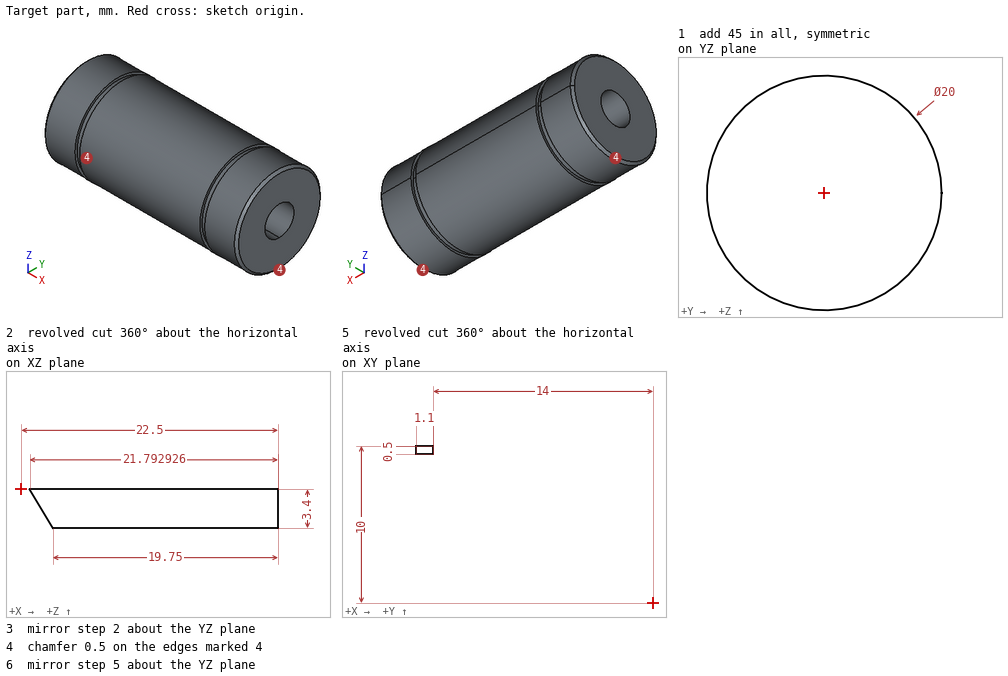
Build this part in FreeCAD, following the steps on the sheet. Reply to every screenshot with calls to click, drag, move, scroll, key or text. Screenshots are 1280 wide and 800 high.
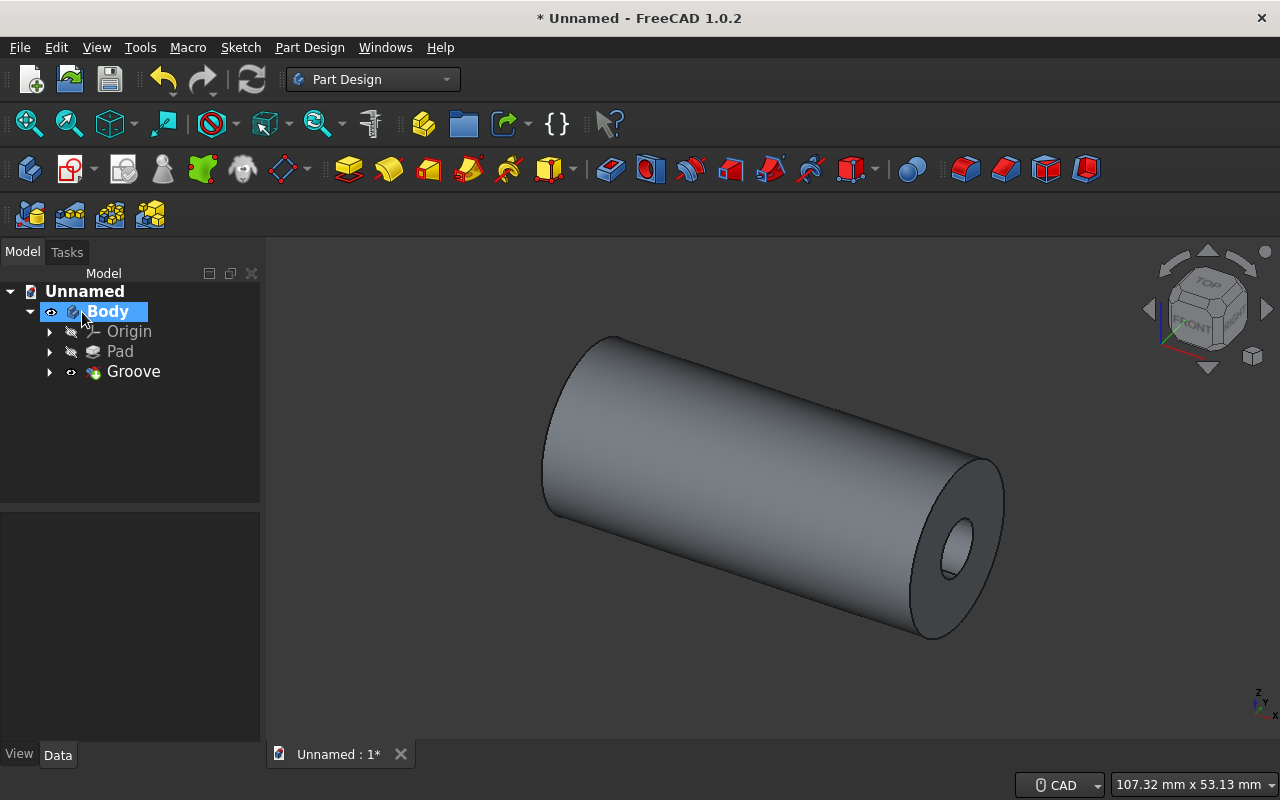
click(116, 372)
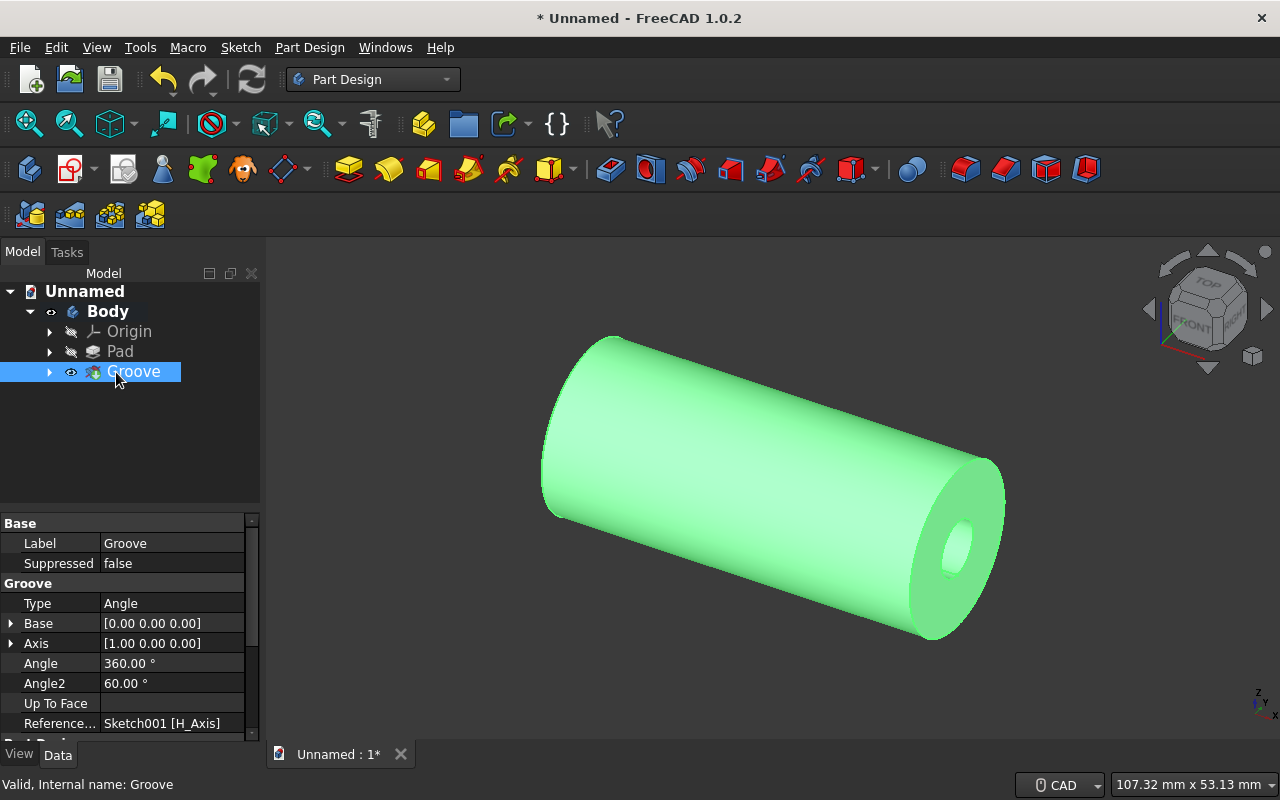
click(30, 214)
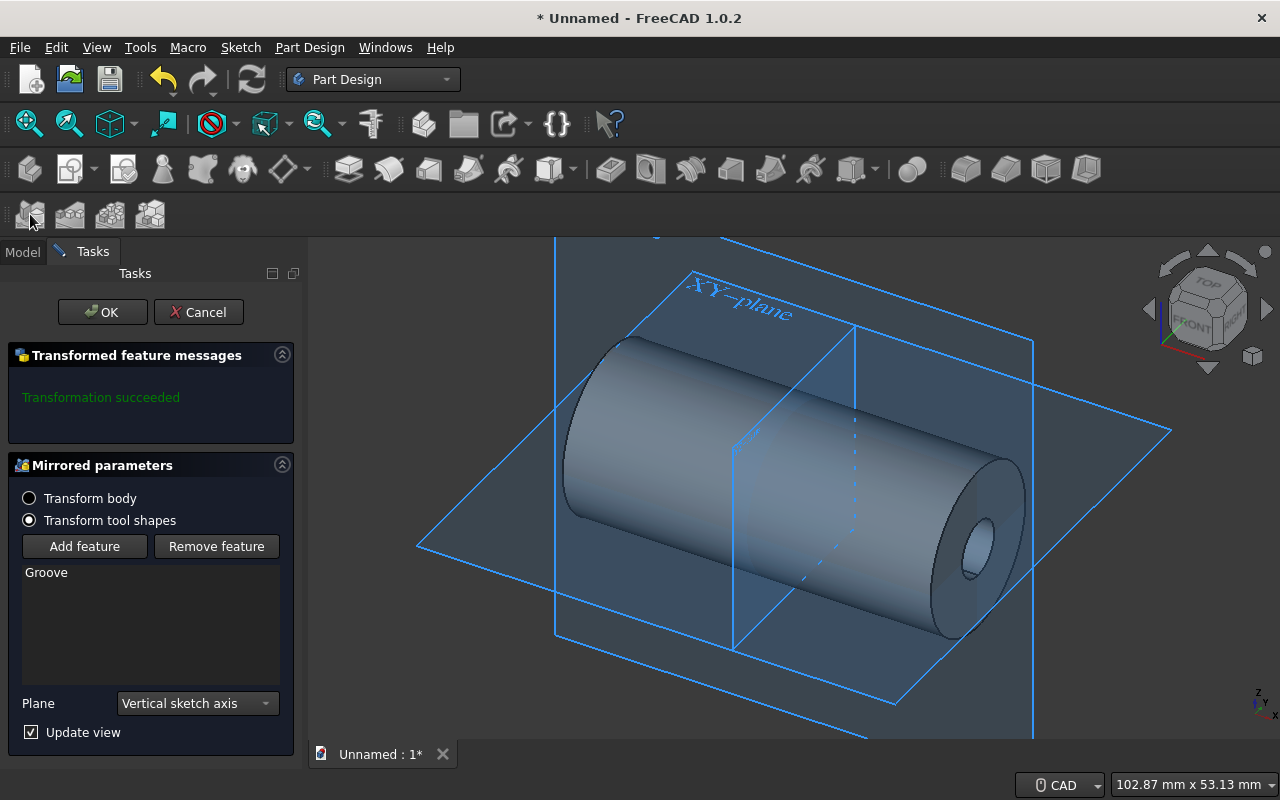
click(198, 704)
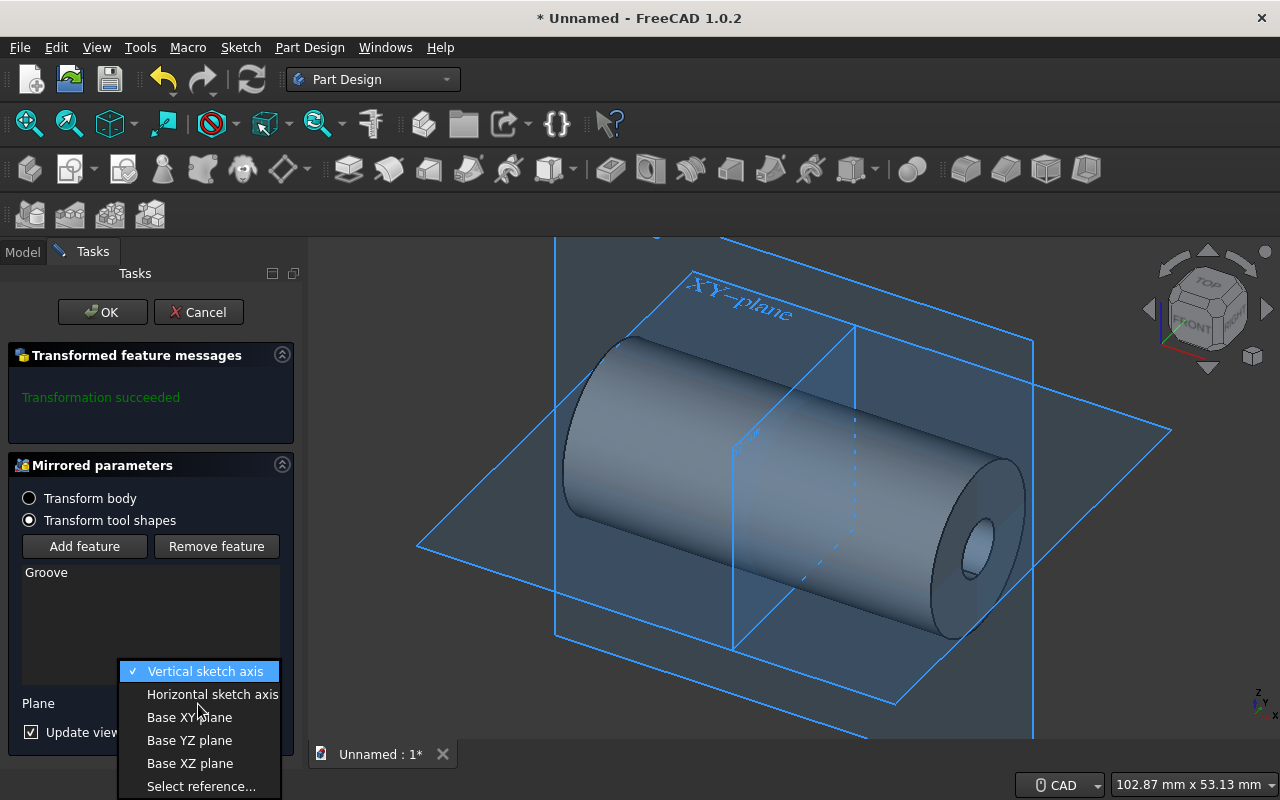
click(198, 740)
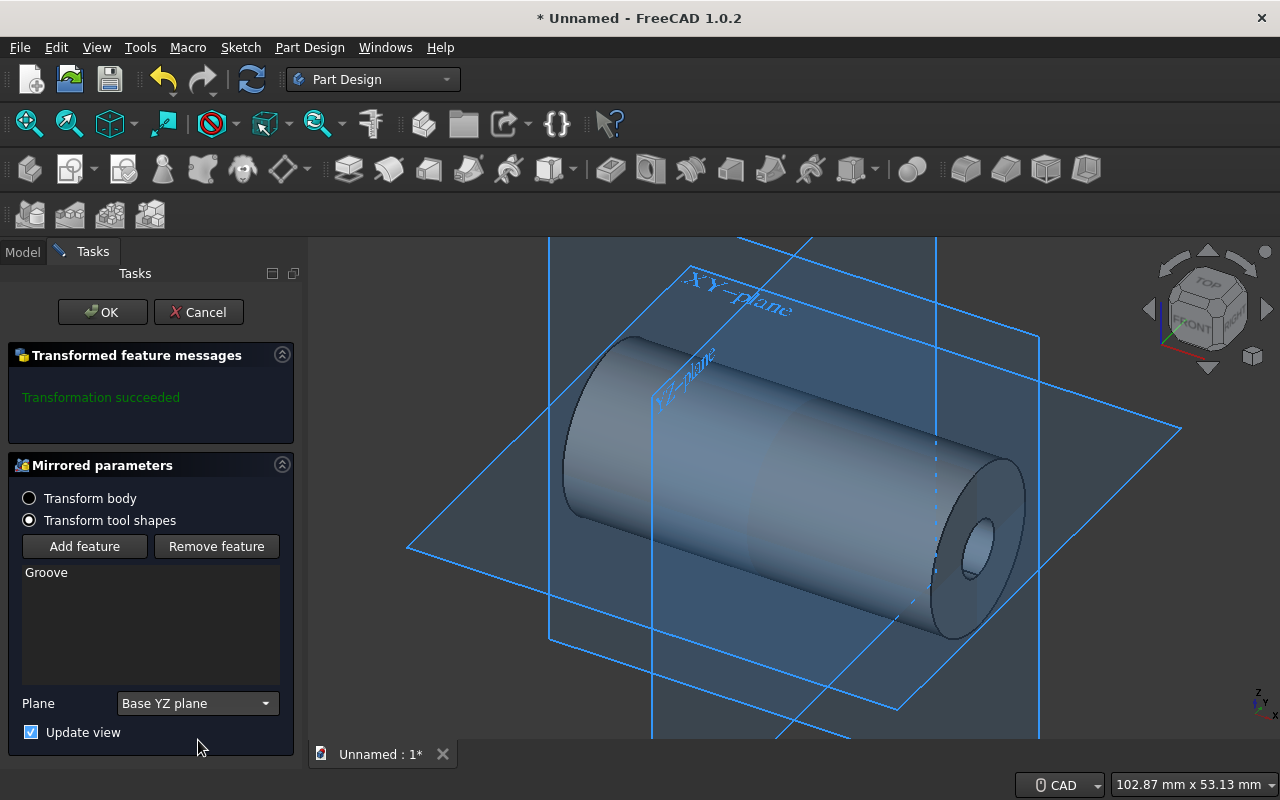
click(103, 312)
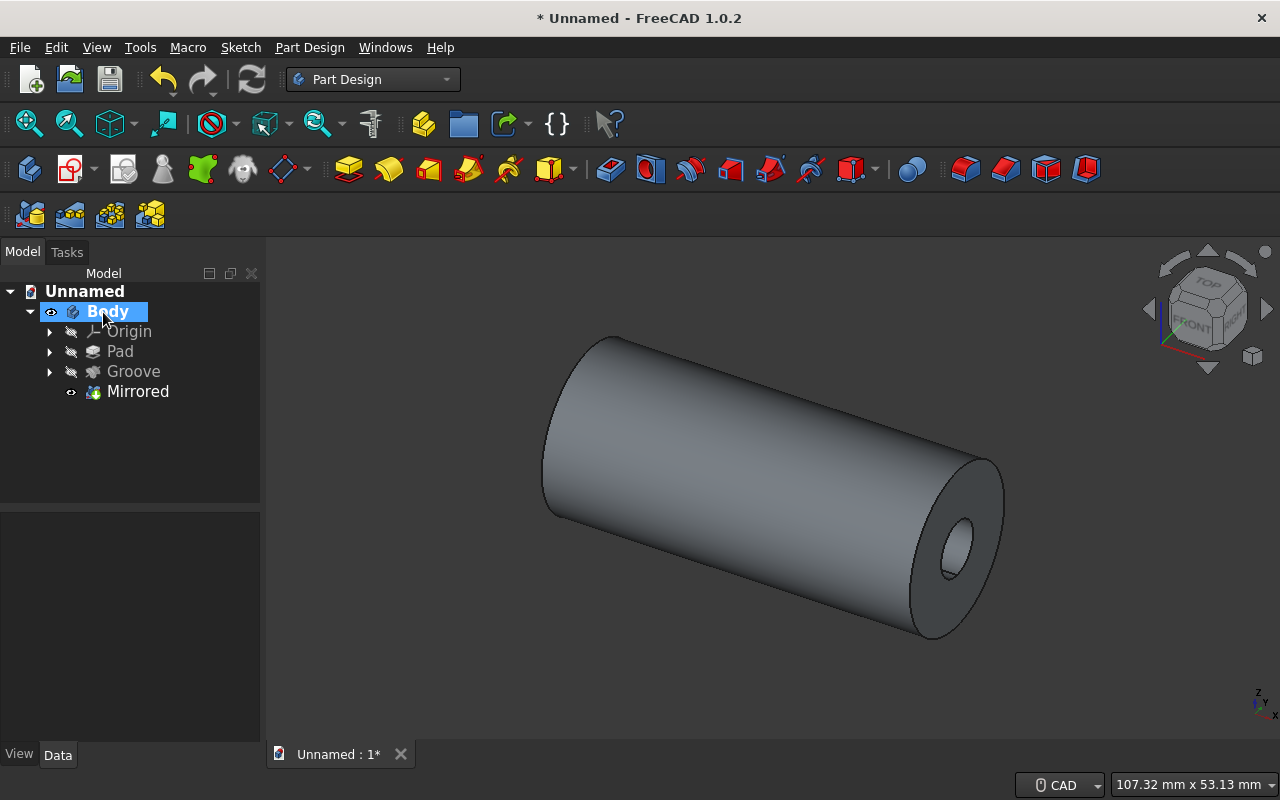
click(574, 367)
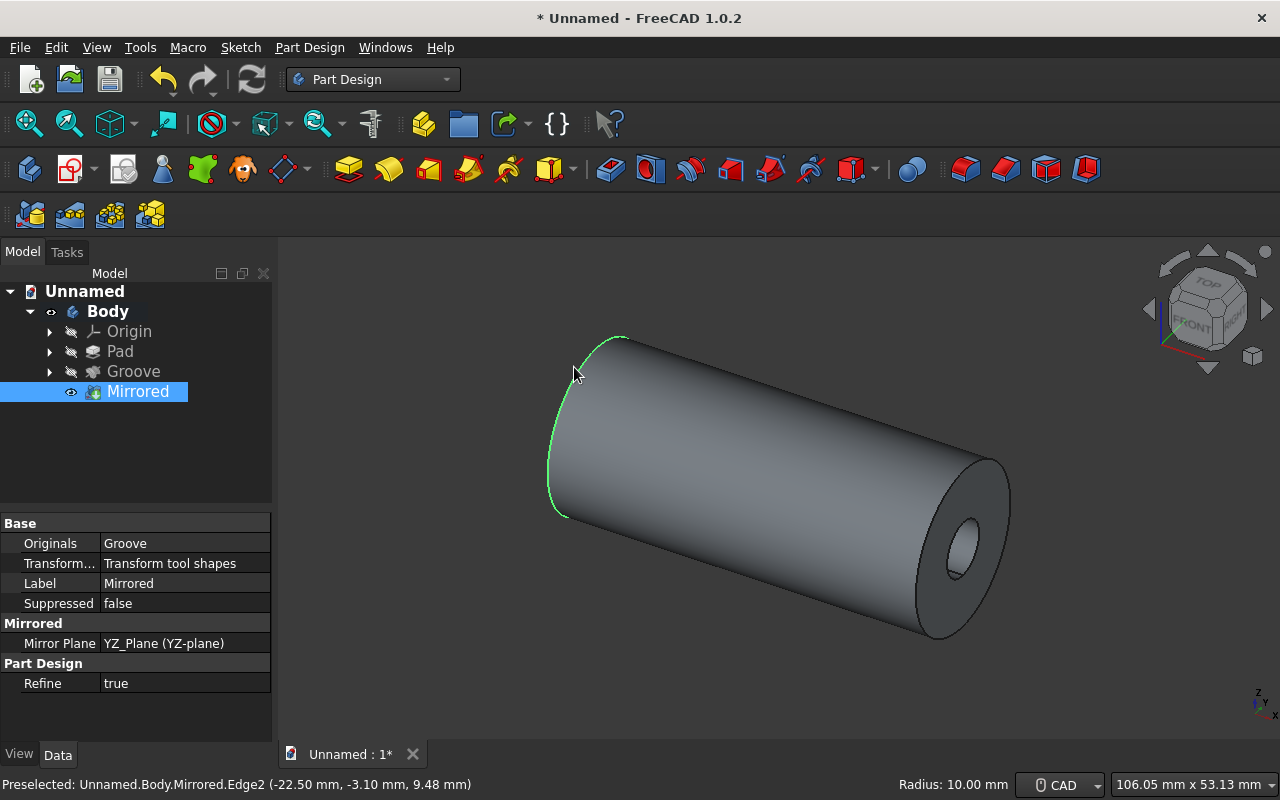
click(916, 595, ctrl)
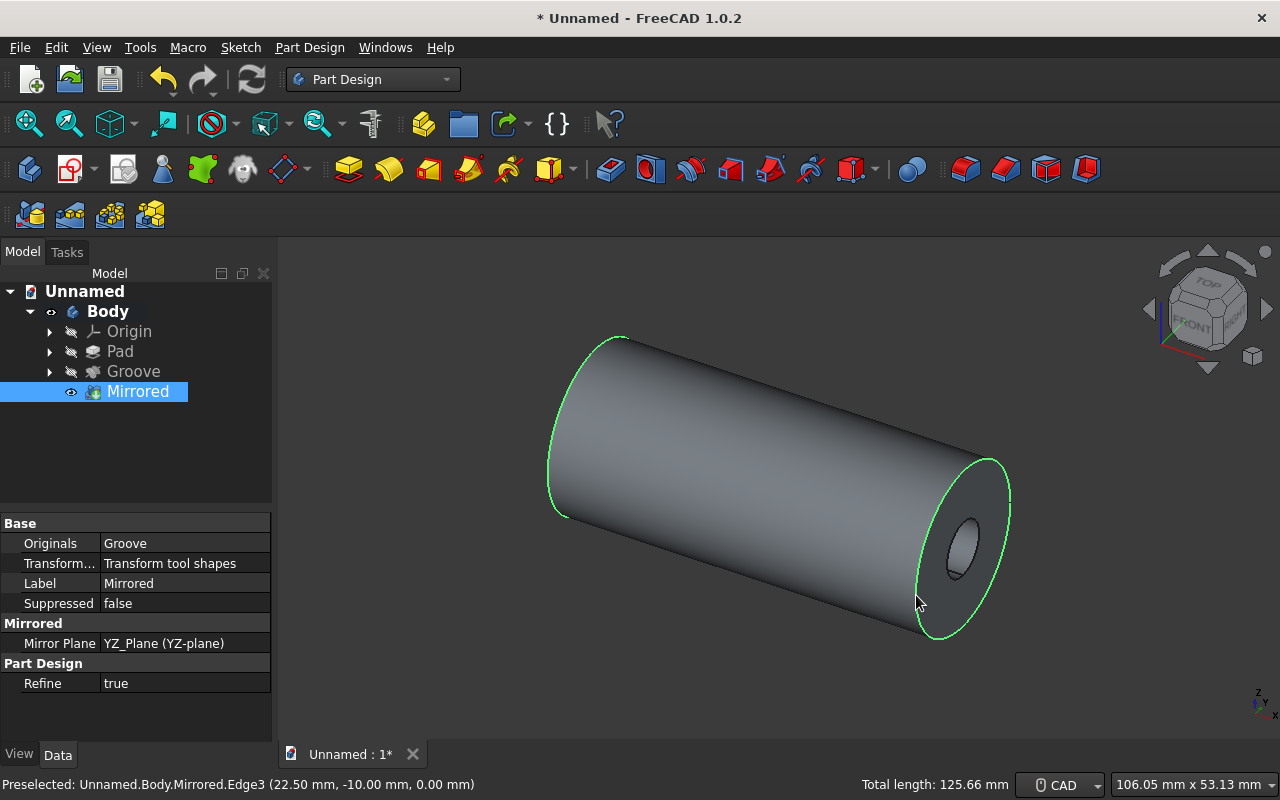
click(1006, 170)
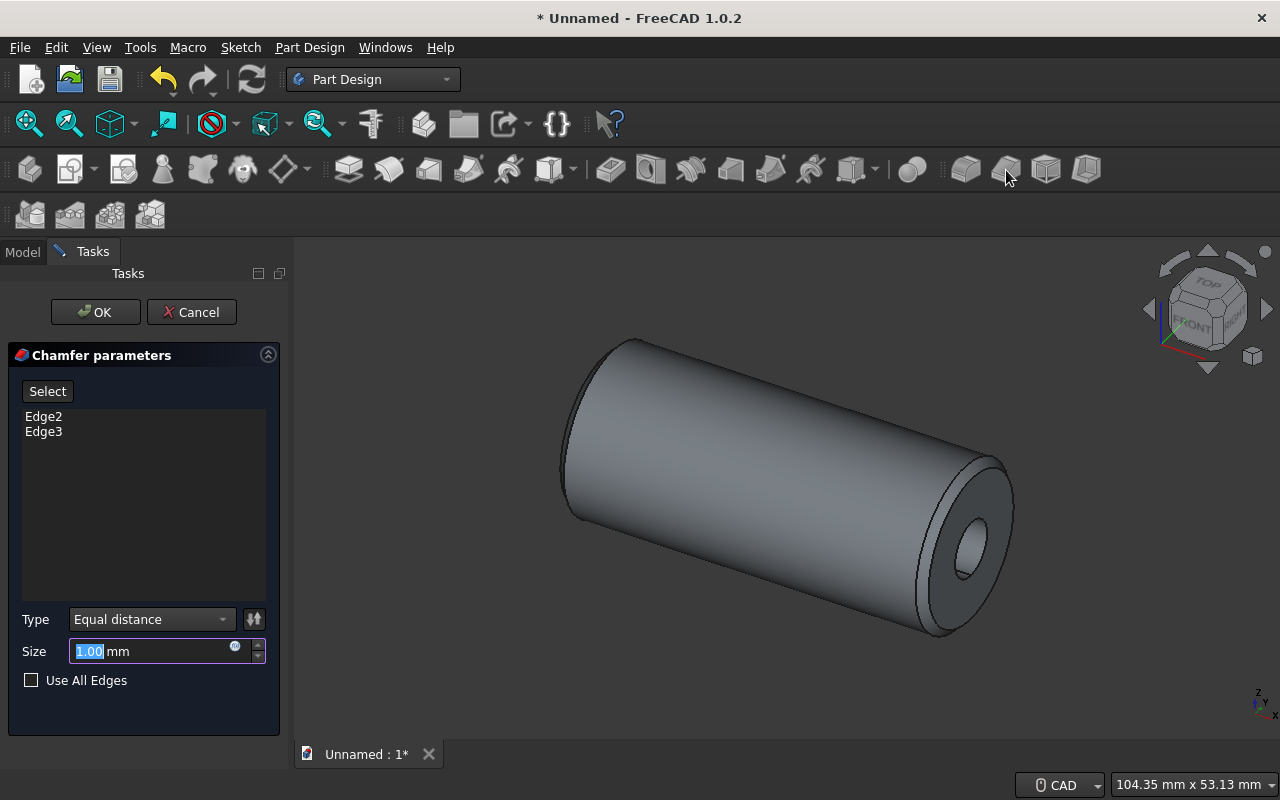
text(0.5)
key(Tab)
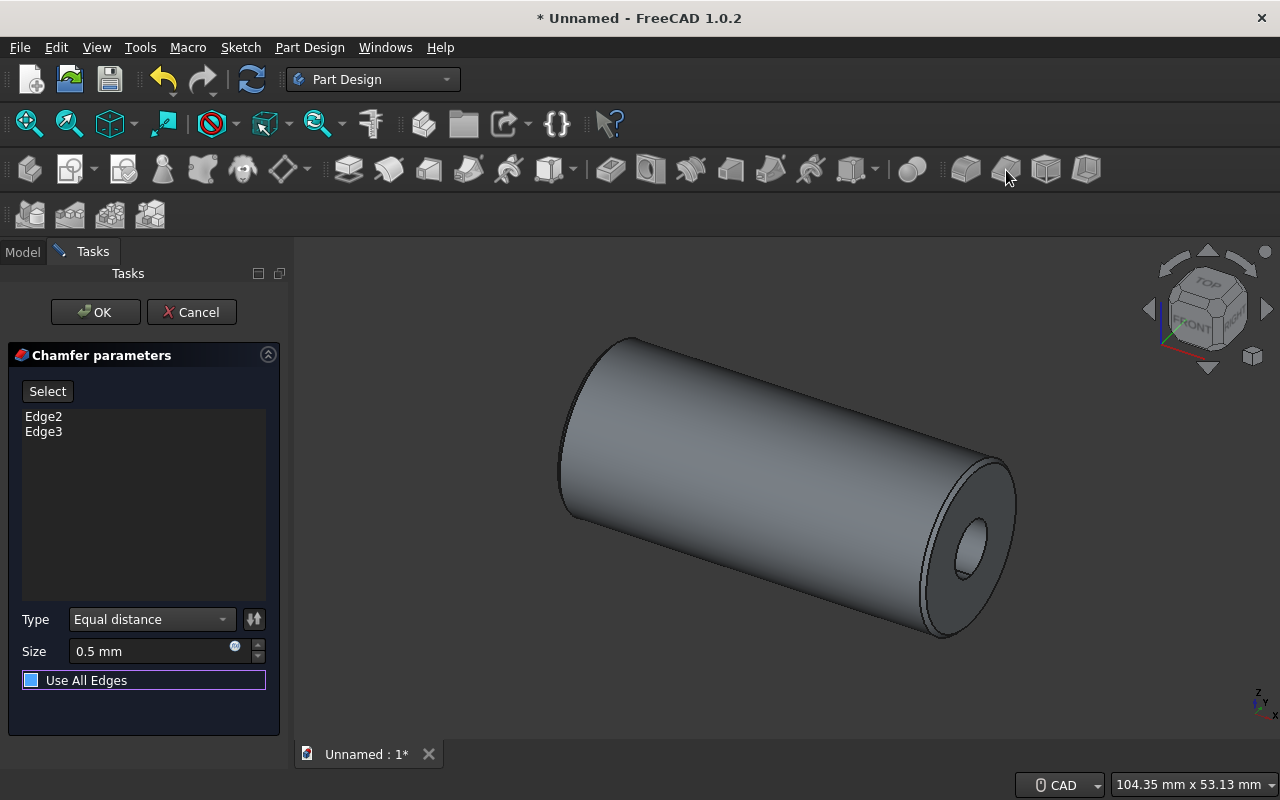
click(96, 312)